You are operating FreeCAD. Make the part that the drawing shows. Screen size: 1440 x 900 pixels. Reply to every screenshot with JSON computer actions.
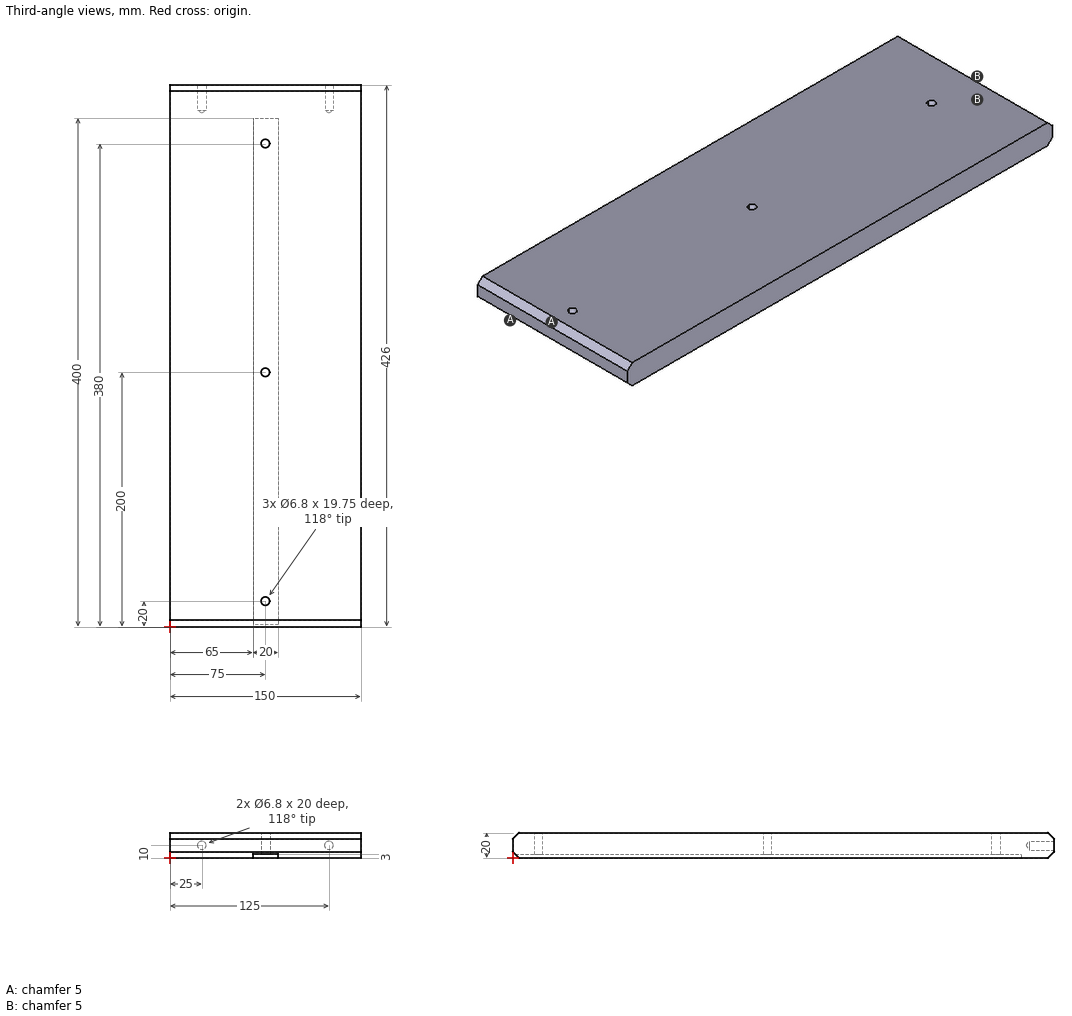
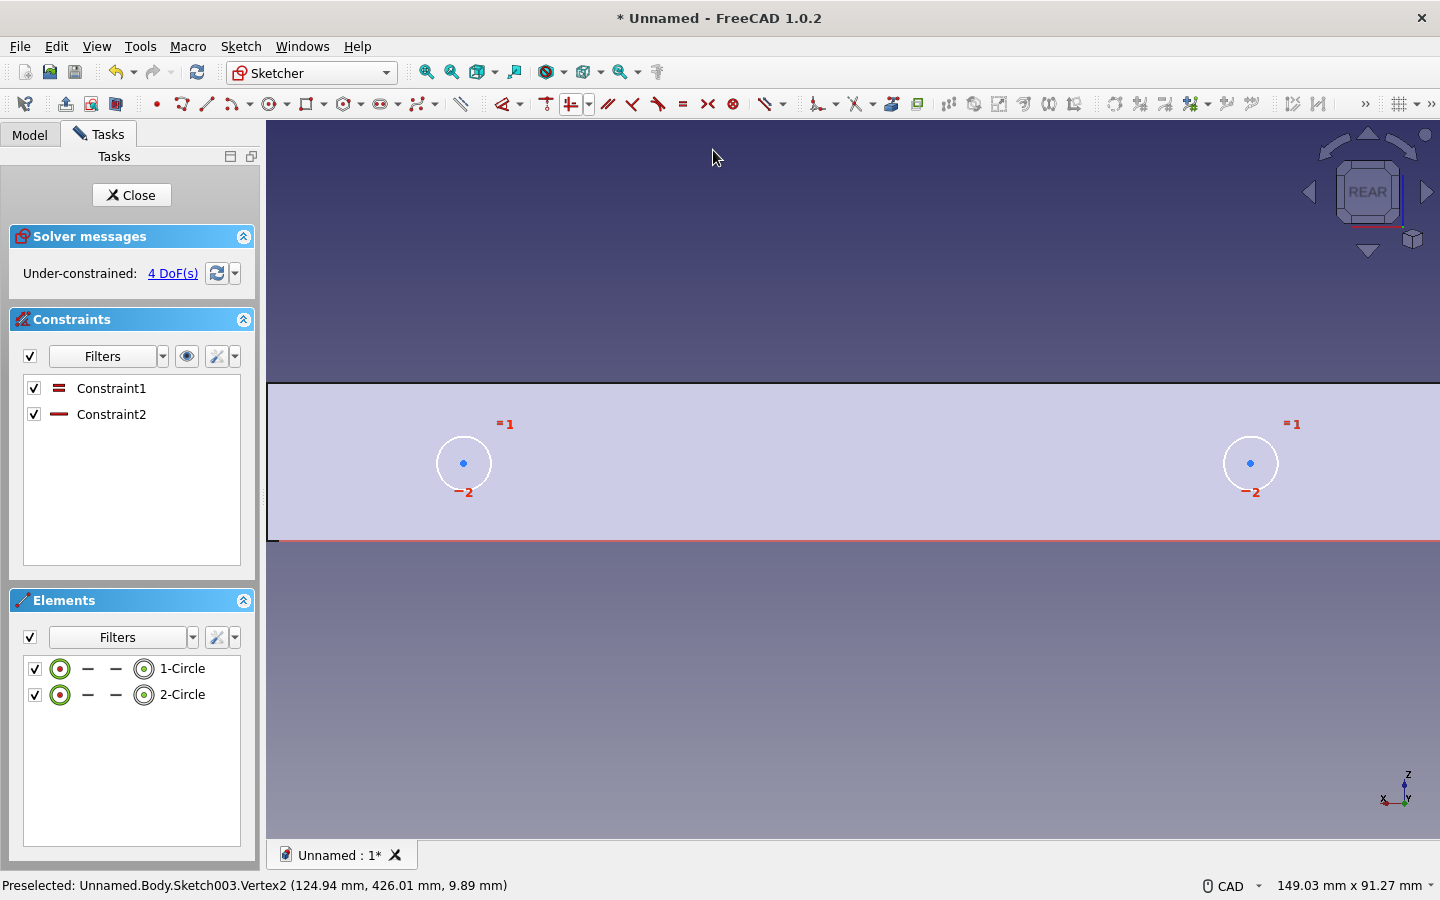
{"action": "key", "text": "d"}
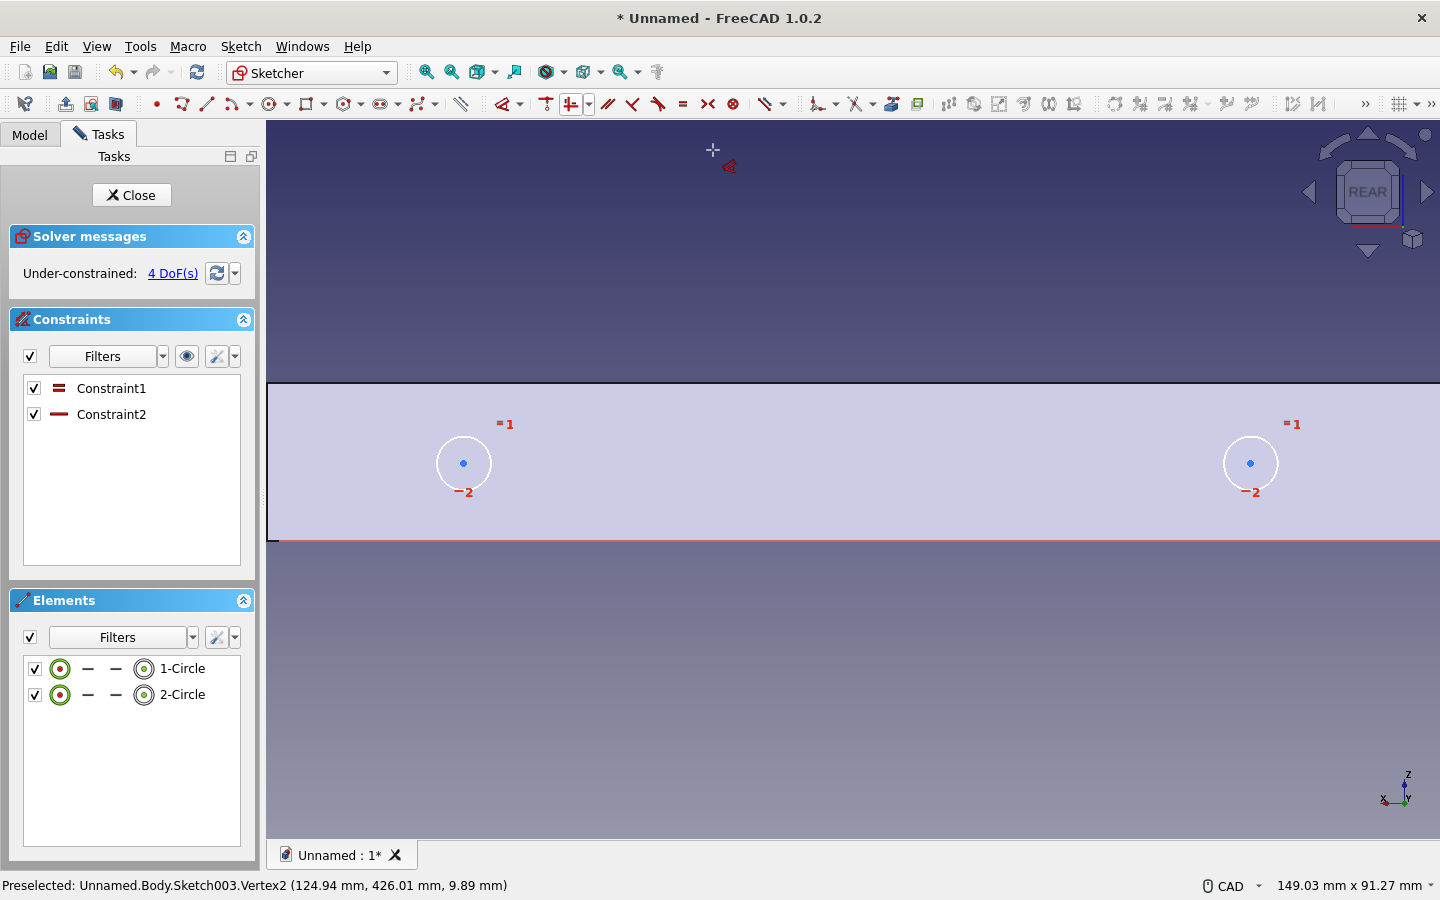
{"action": "left_click", "coordinate": [1270, 444]}
{"action": "left_click", "coordinate": [1267, 406]}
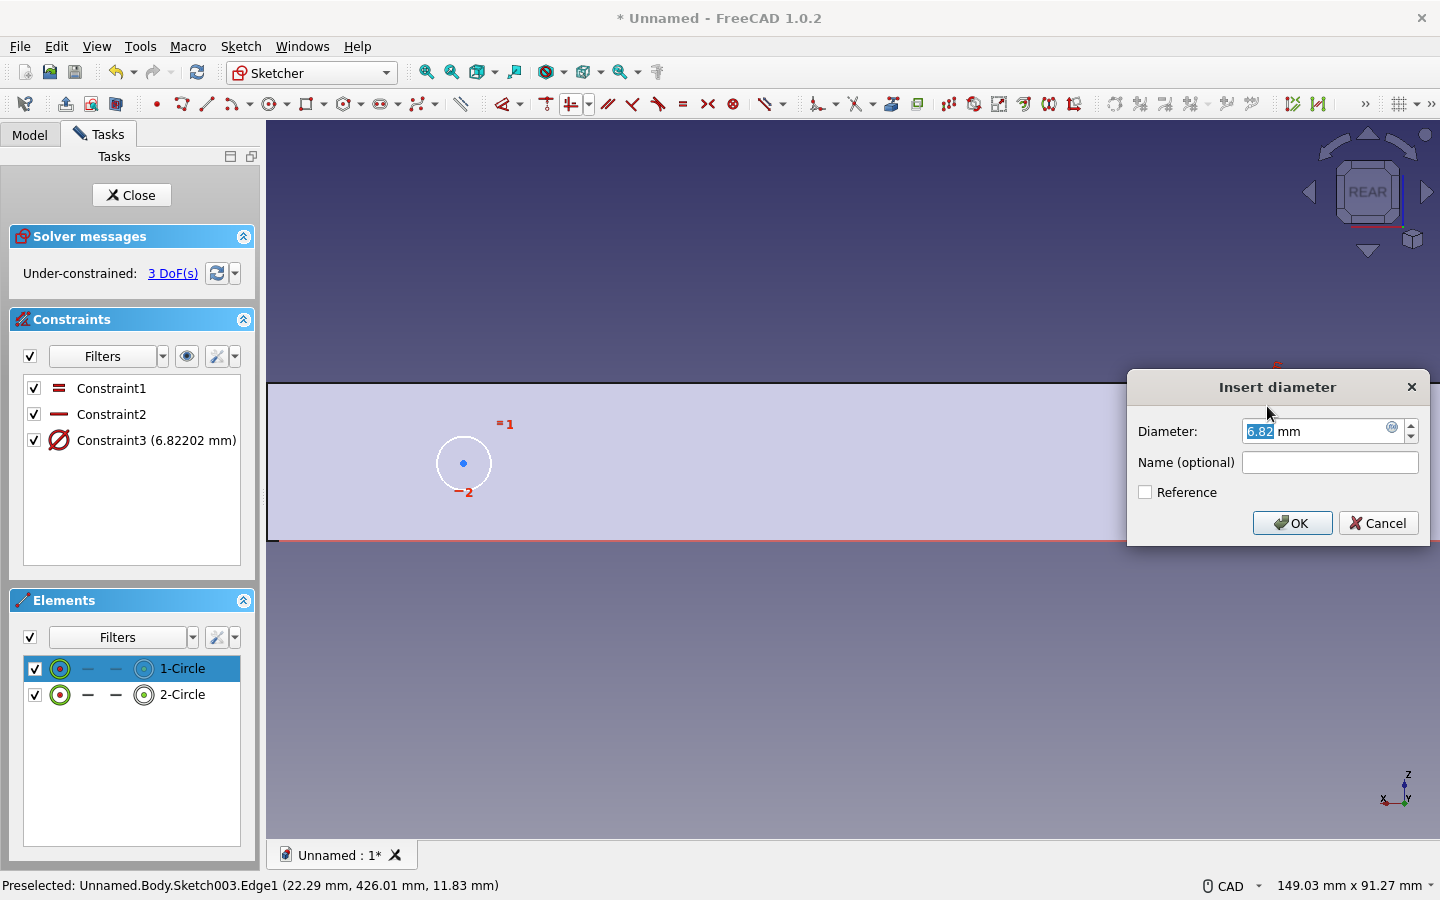
{"action": "type", "text": "6.8"}
{"action": "key", "text": "Return"}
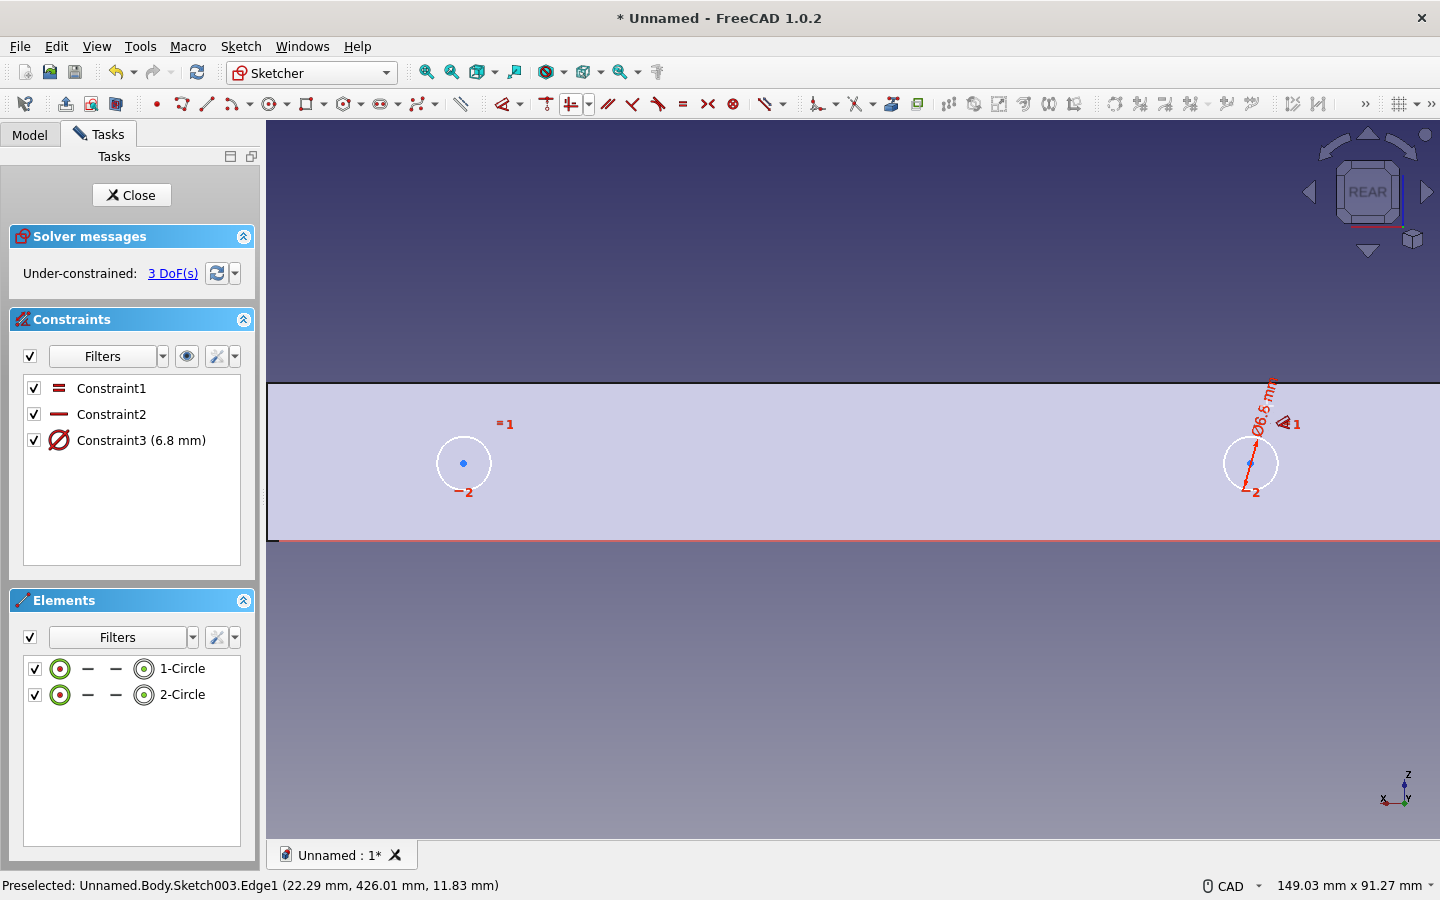
{"action": "left_click", "coordinate": [1251, 463]}
{"action": "left_click", "coordinate": [1263, 575]}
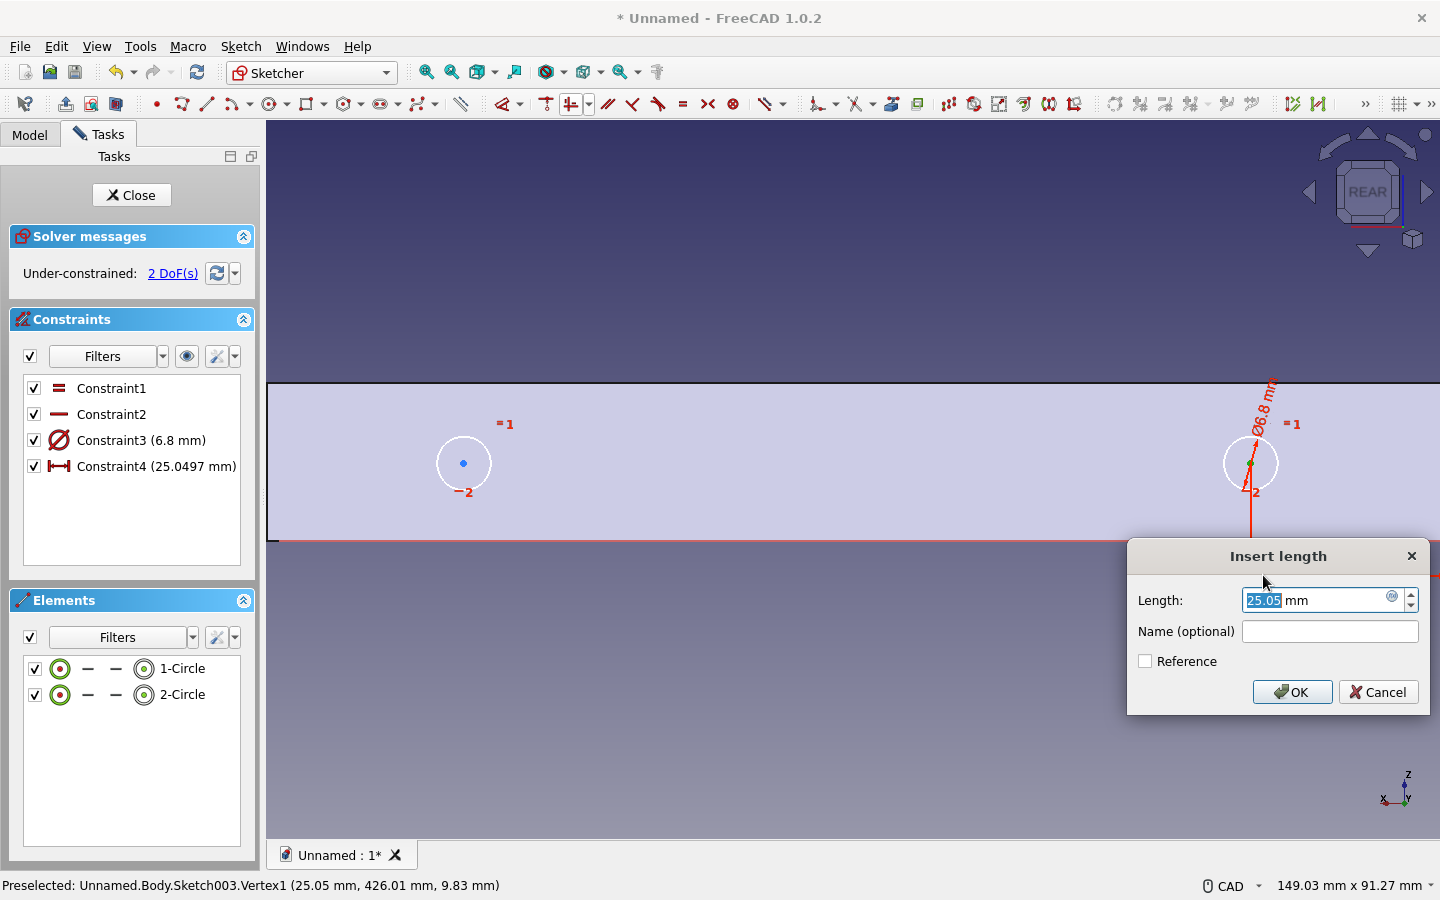
{"action": "type", "text": "25"}
{"action": "key", "text": "Return"}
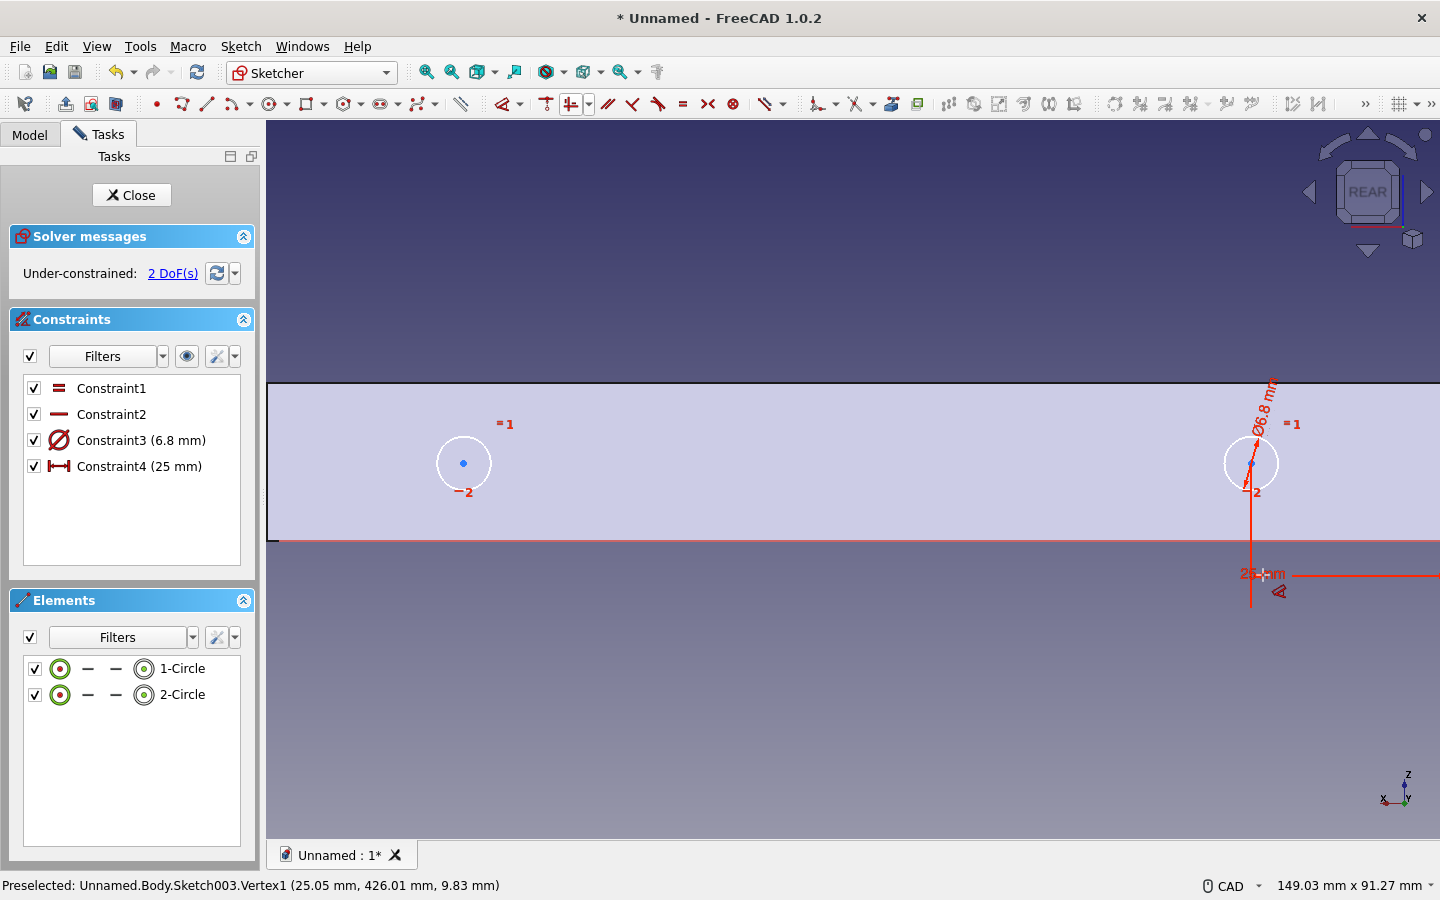
{"action": "left_click", "coordinate": [1251, 463]}
{"action": "left_click", "coordinate": [1217, 502]}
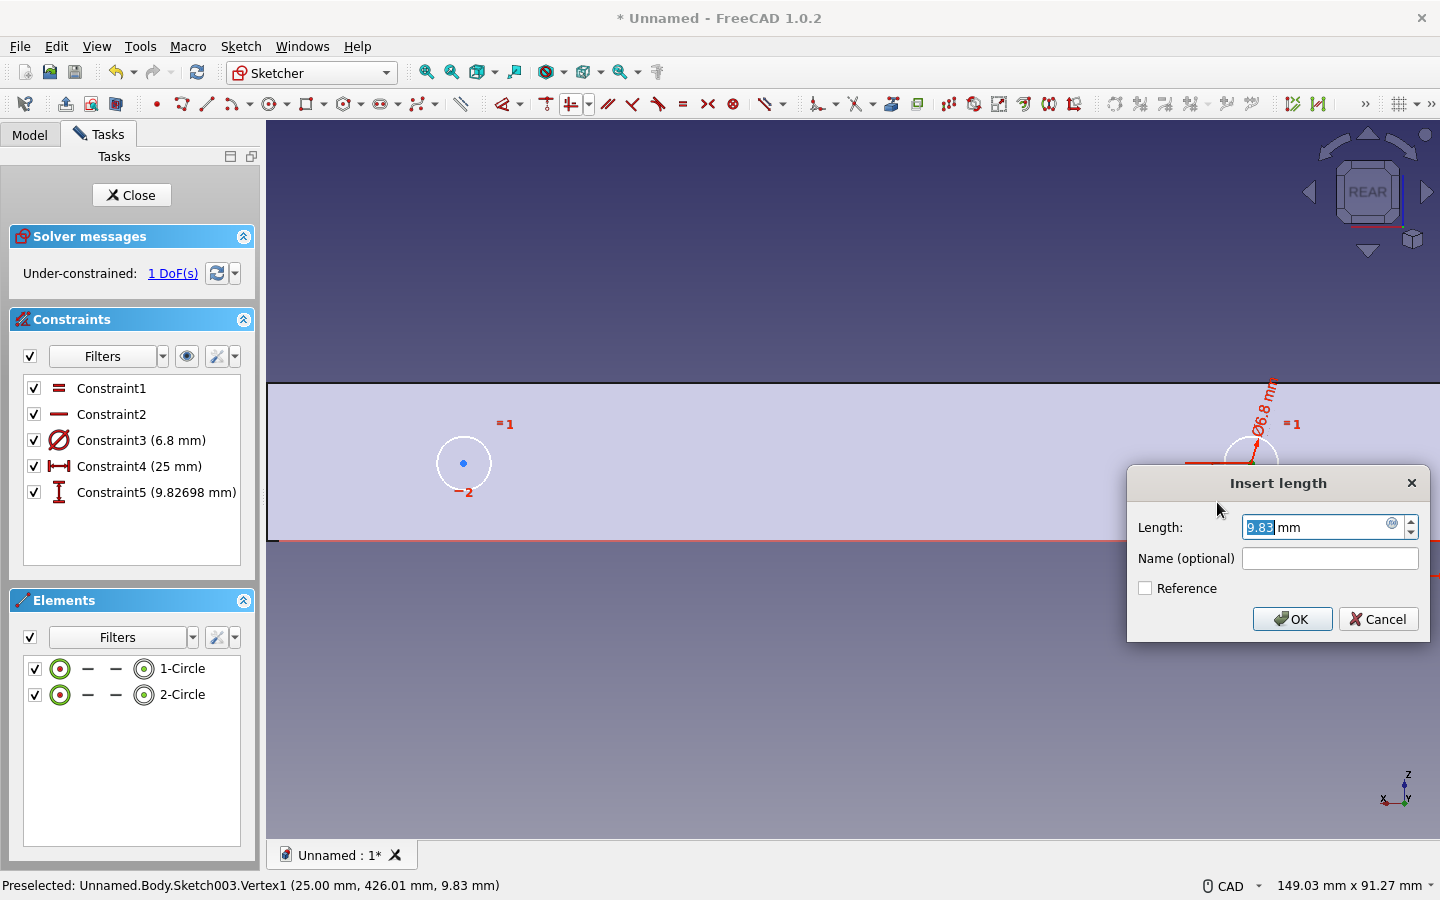
{"action": "type", "text": "10"}
{"action": "key", "text": "Return"}